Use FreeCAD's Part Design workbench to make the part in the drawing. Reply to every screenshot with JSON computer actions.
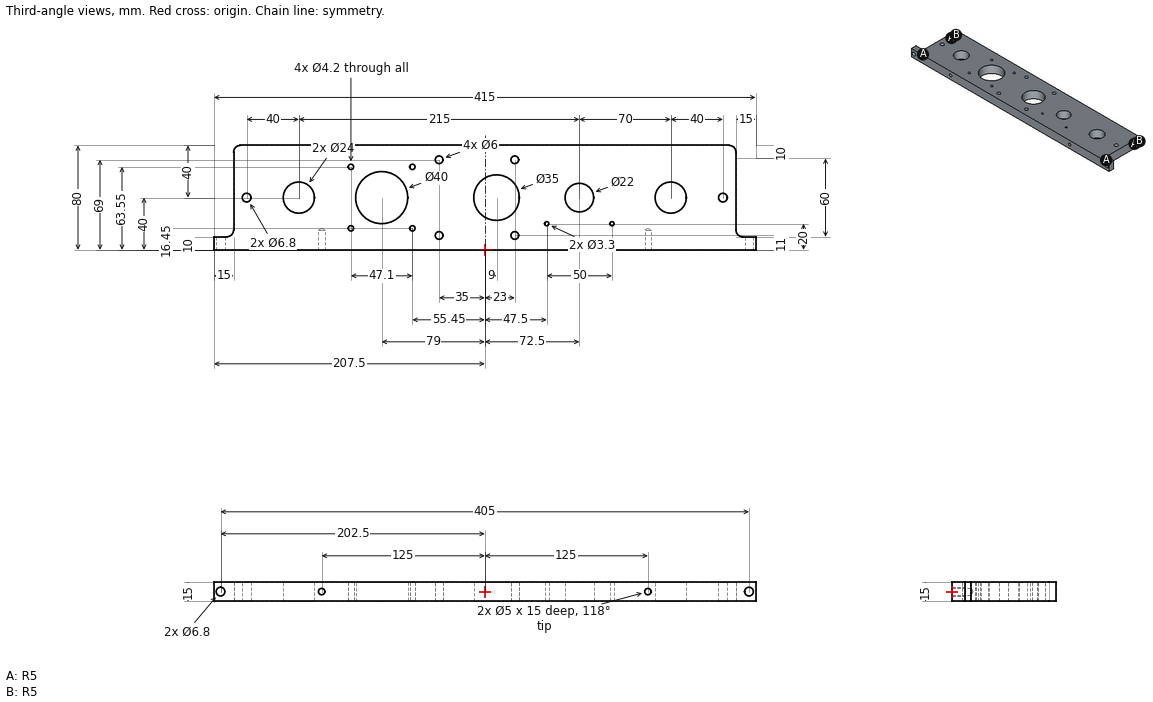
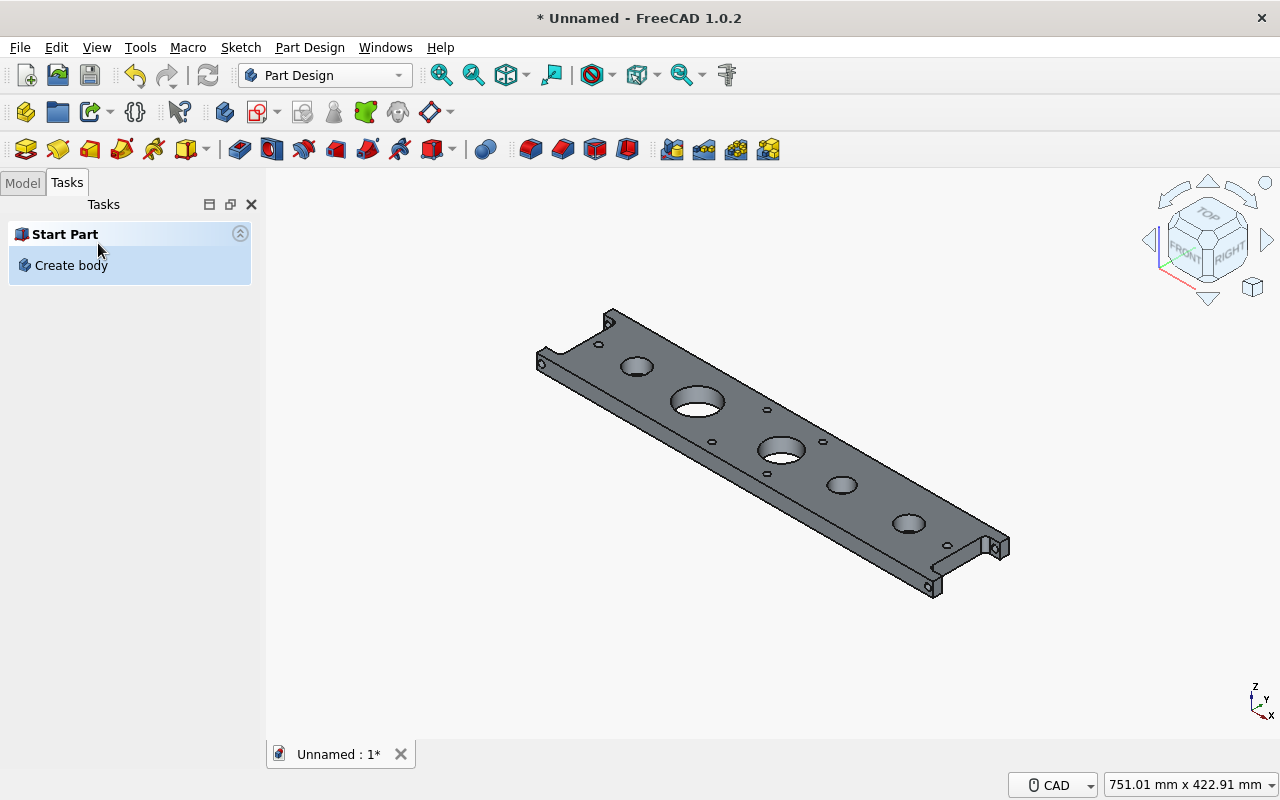
{"action": "left_click", "coordinate": [908, 497]}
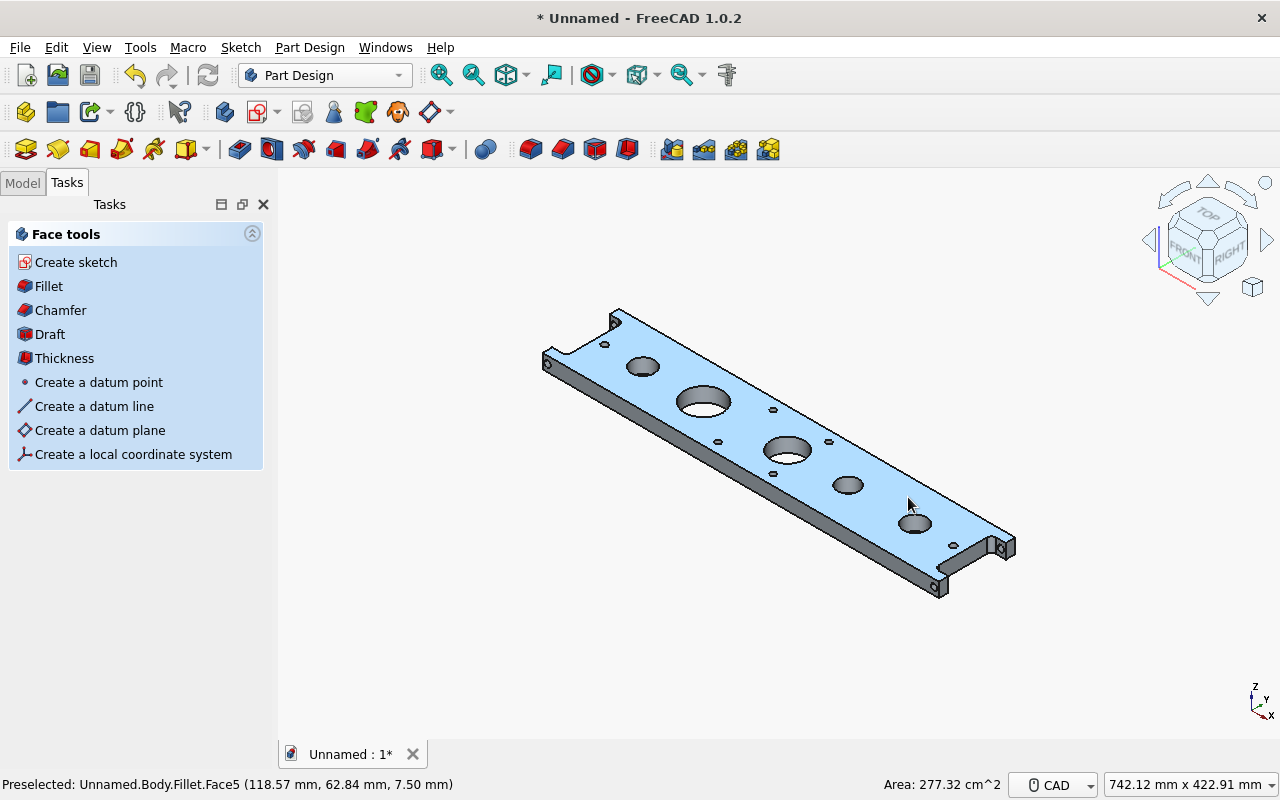
{"action": "left_click", "coordinate": [258, 112]}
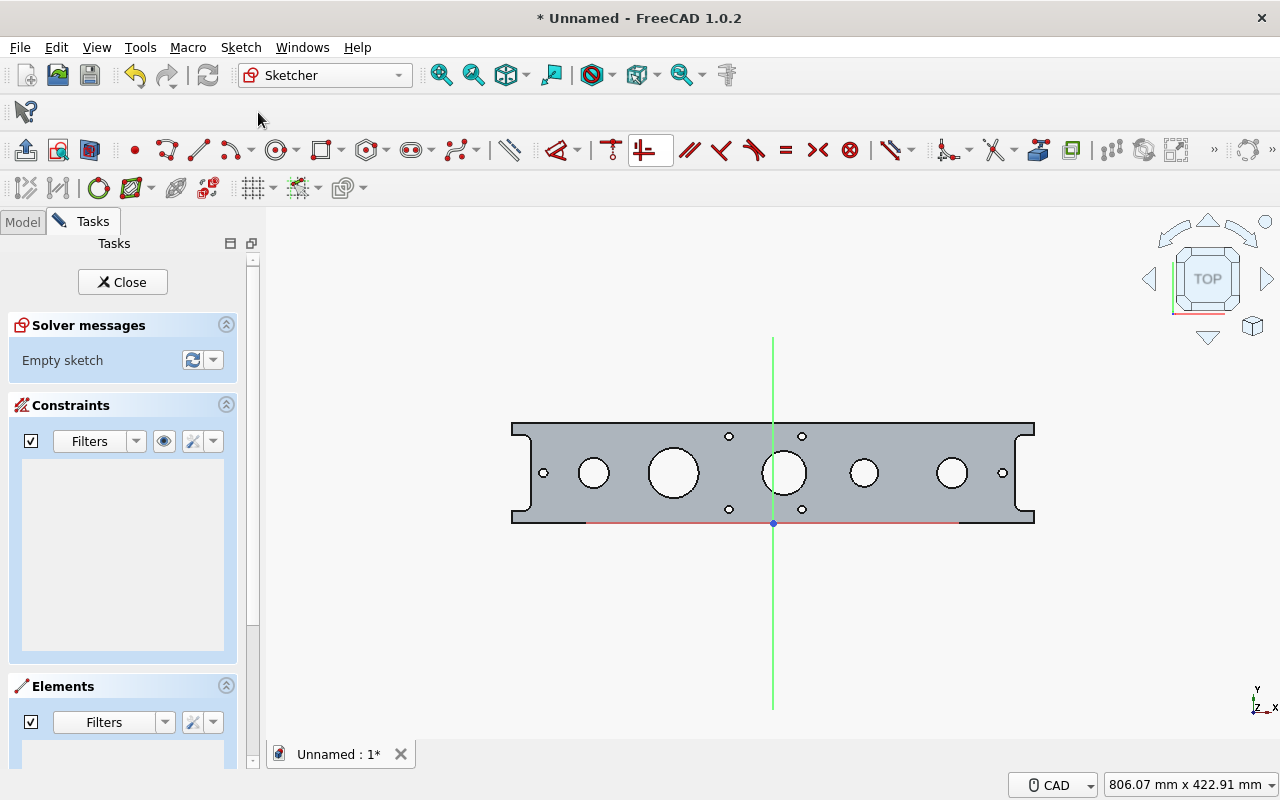
{"action": "scroll", "coordinate": [868, 519], "scroll_direction": "up", "scroll_amount": 8}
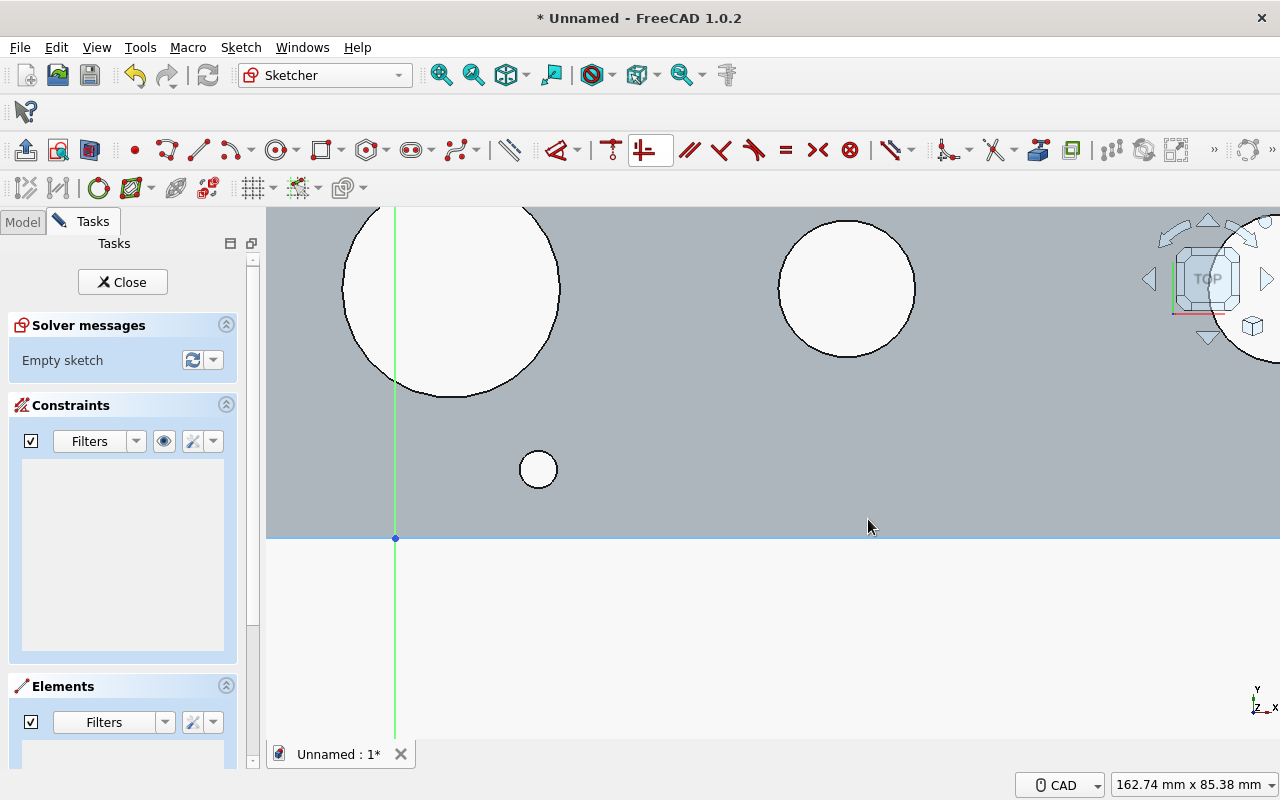
{"action": "left_click", "coordinate": [276, 150]}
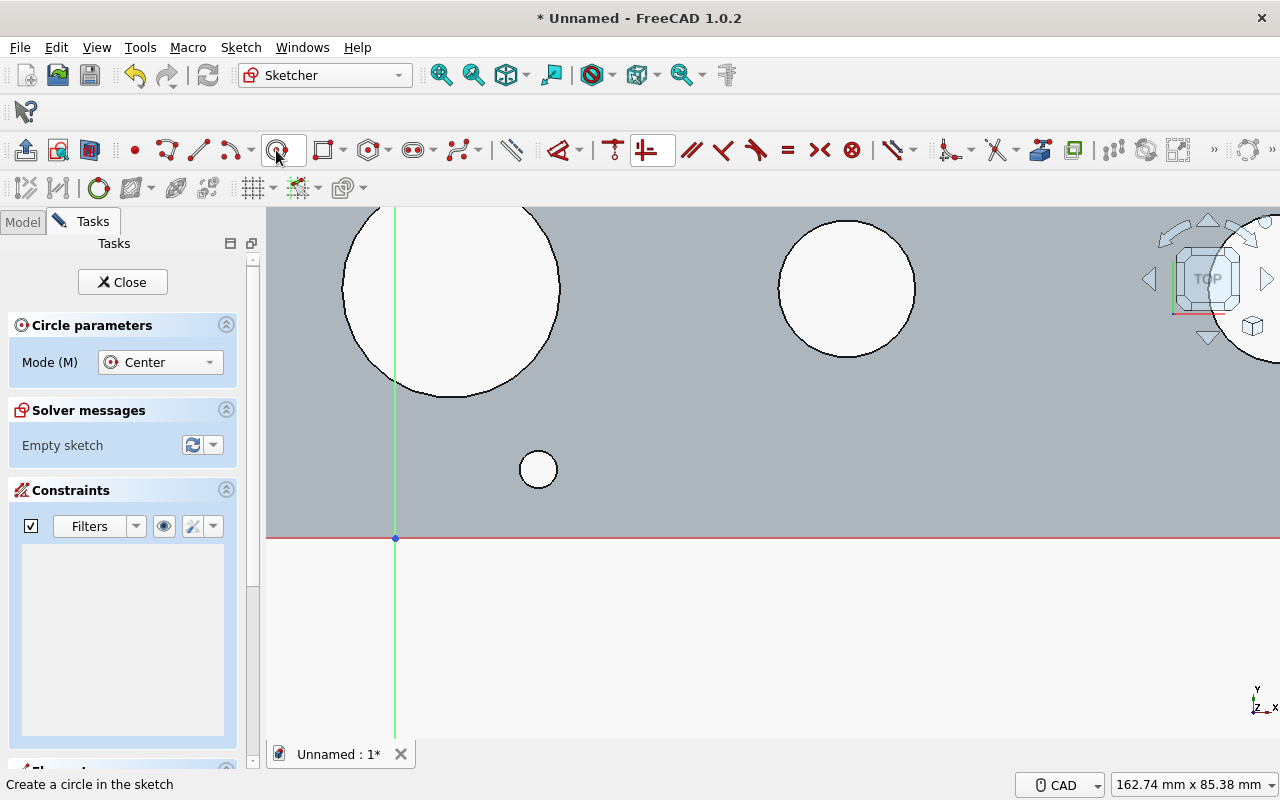
{"action": "scroll", "coordinate": [691, 413], "scroll_direction": "up", "scroll_amount": 4}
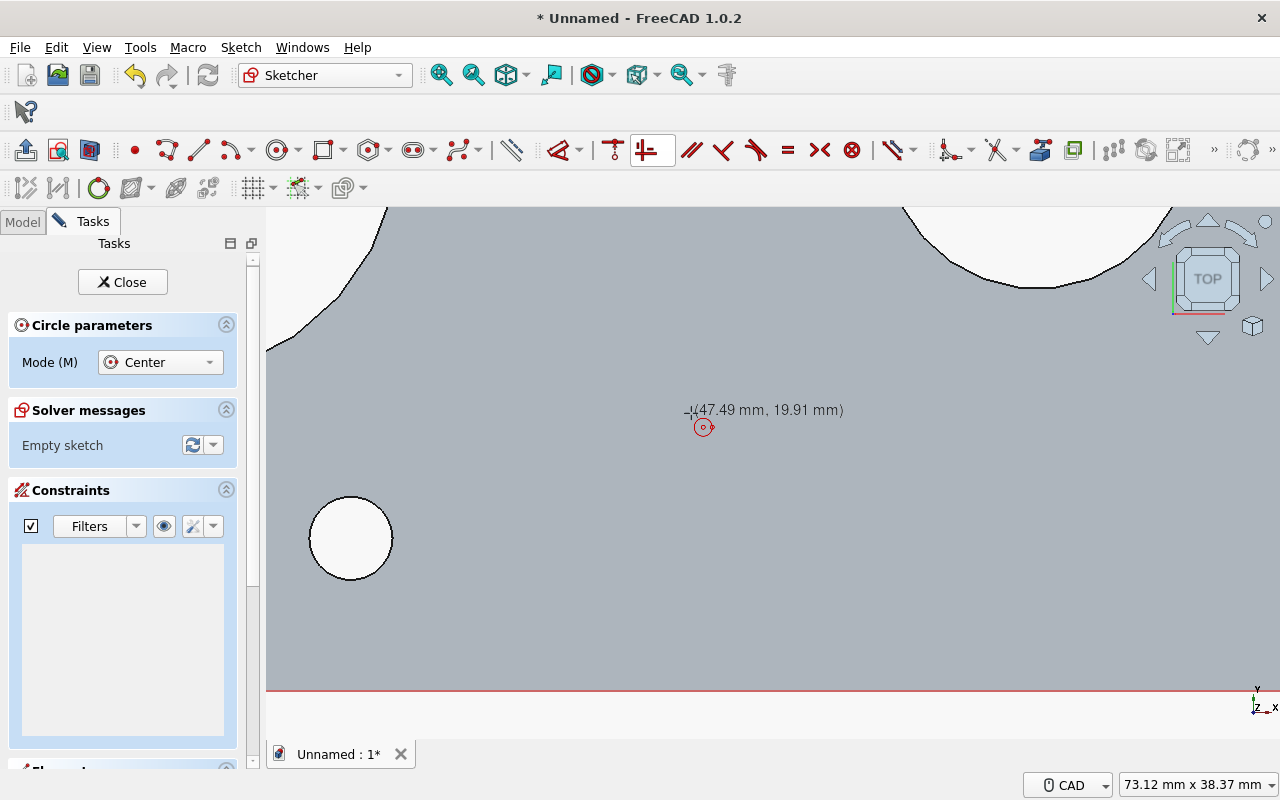
{"action": "left_click", "coordinate": [691, 414]}
{"action": "left_click", "coordinate": [707, 397]}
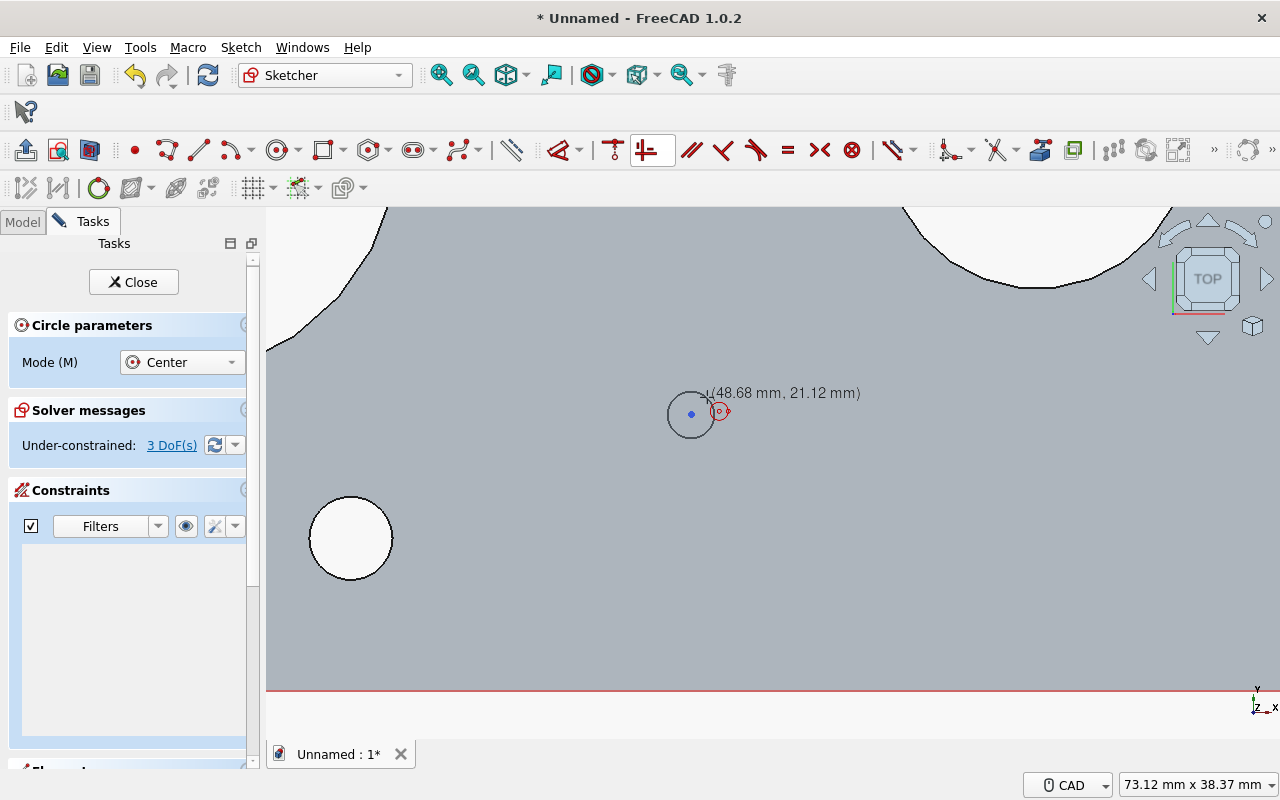
{"action": "scroll", "coordinate": [692, 418], "scroll_direction": "down", "scroll_amount": 4}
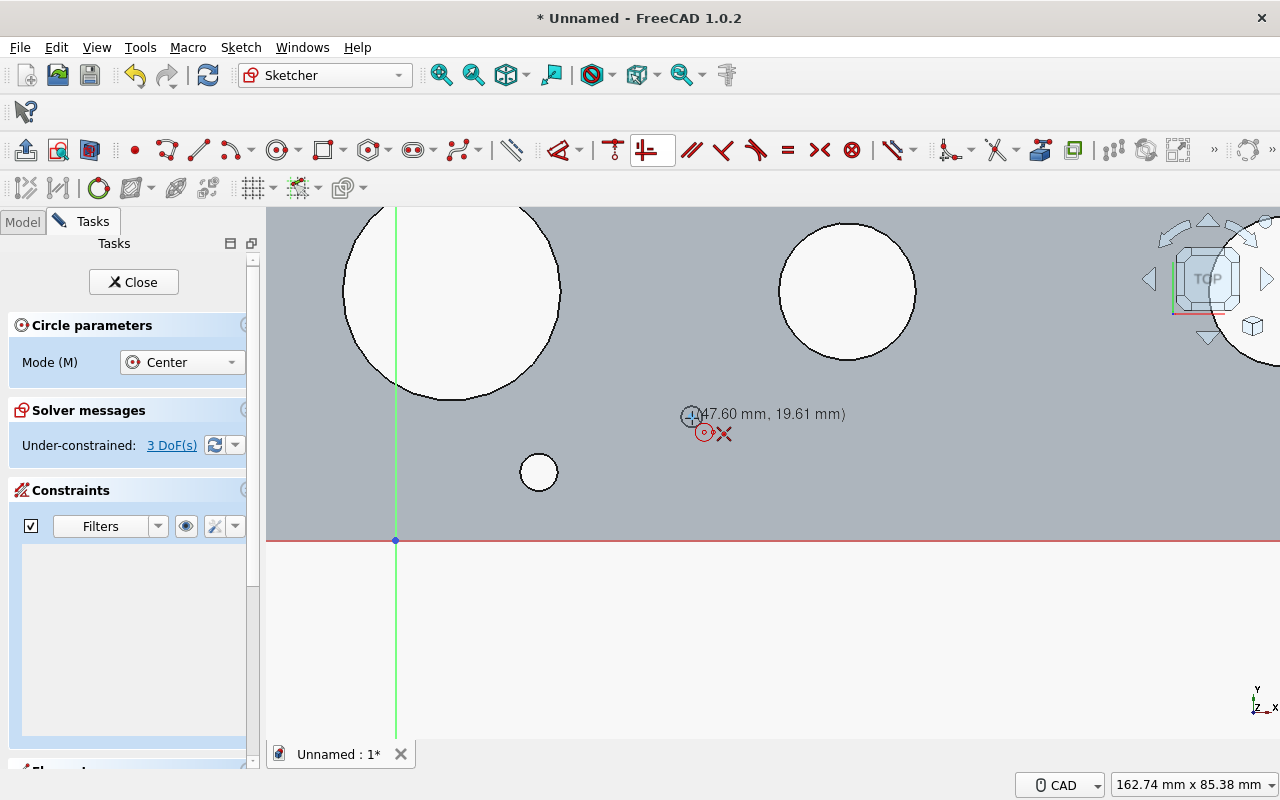
{"action": "scroll", "coordinate": [1003, 416], "scroll_direction": "up", "scroll_amount": 4}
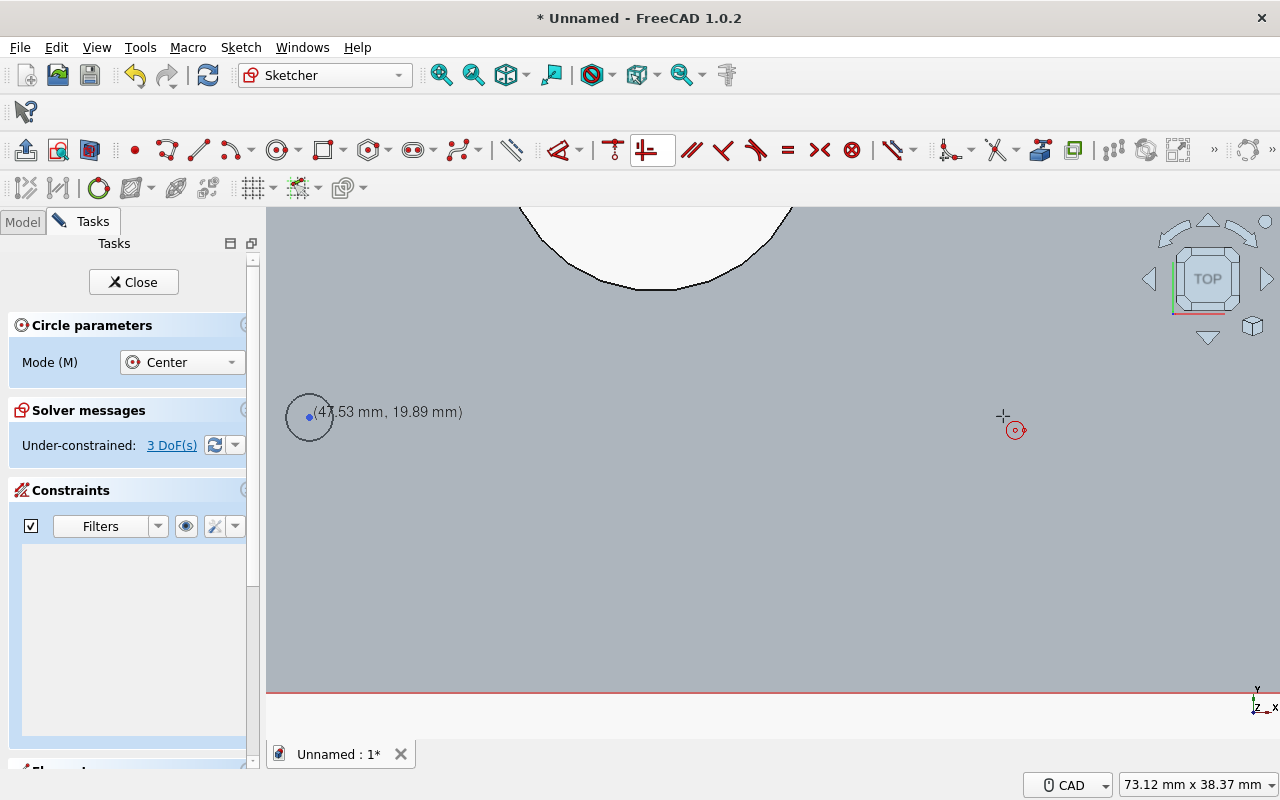
{"action": "left_click", "coordinate": [1002, 416]}
{"action": "left_click", "coordinate": [1019, 400]}
{"action": "key", "text": "Escape"}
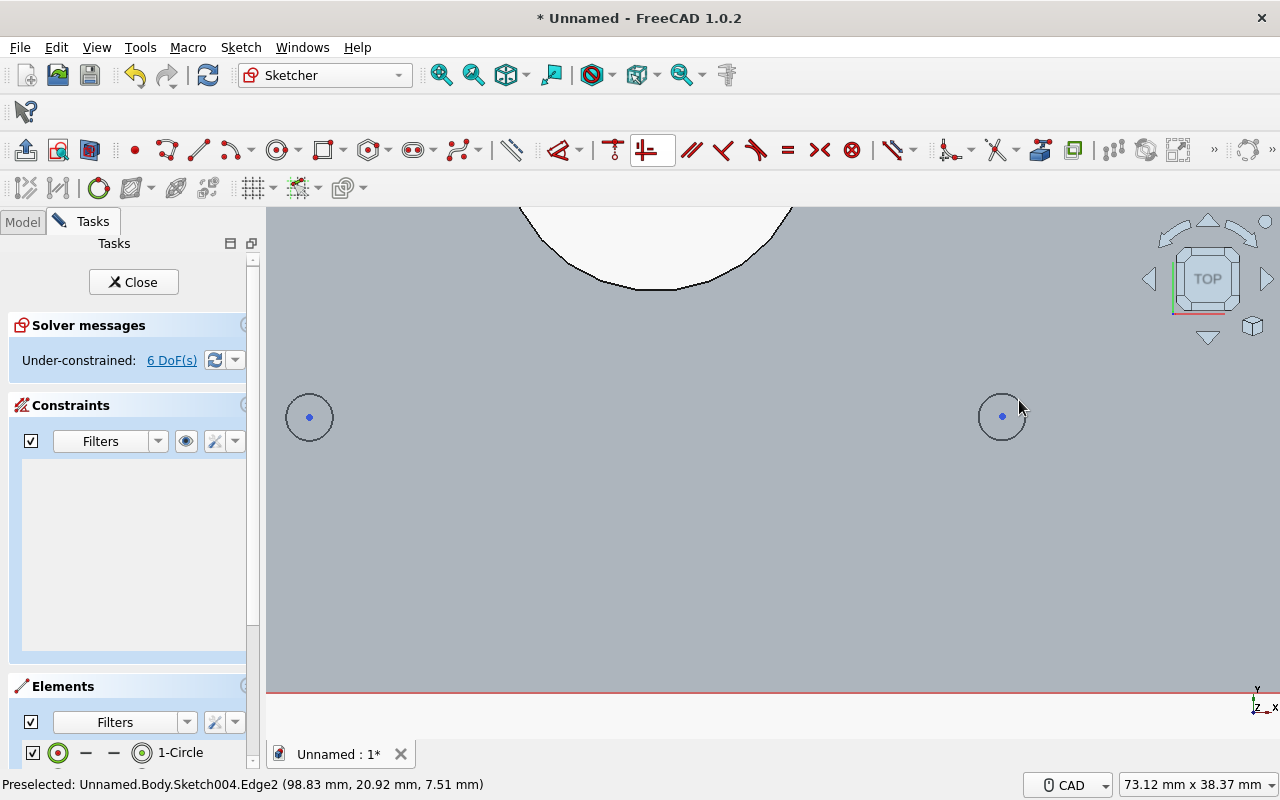
{"action": "left_click", "coordinate": [326, 401]}